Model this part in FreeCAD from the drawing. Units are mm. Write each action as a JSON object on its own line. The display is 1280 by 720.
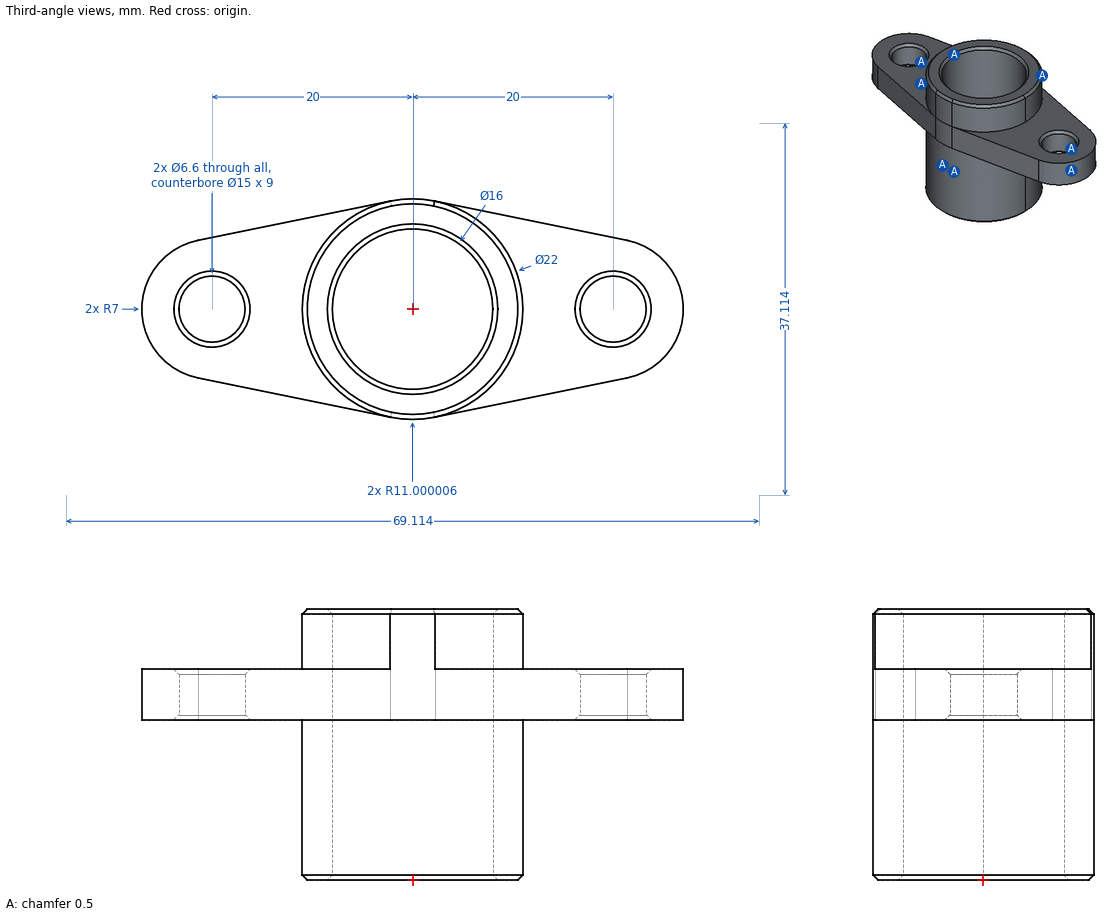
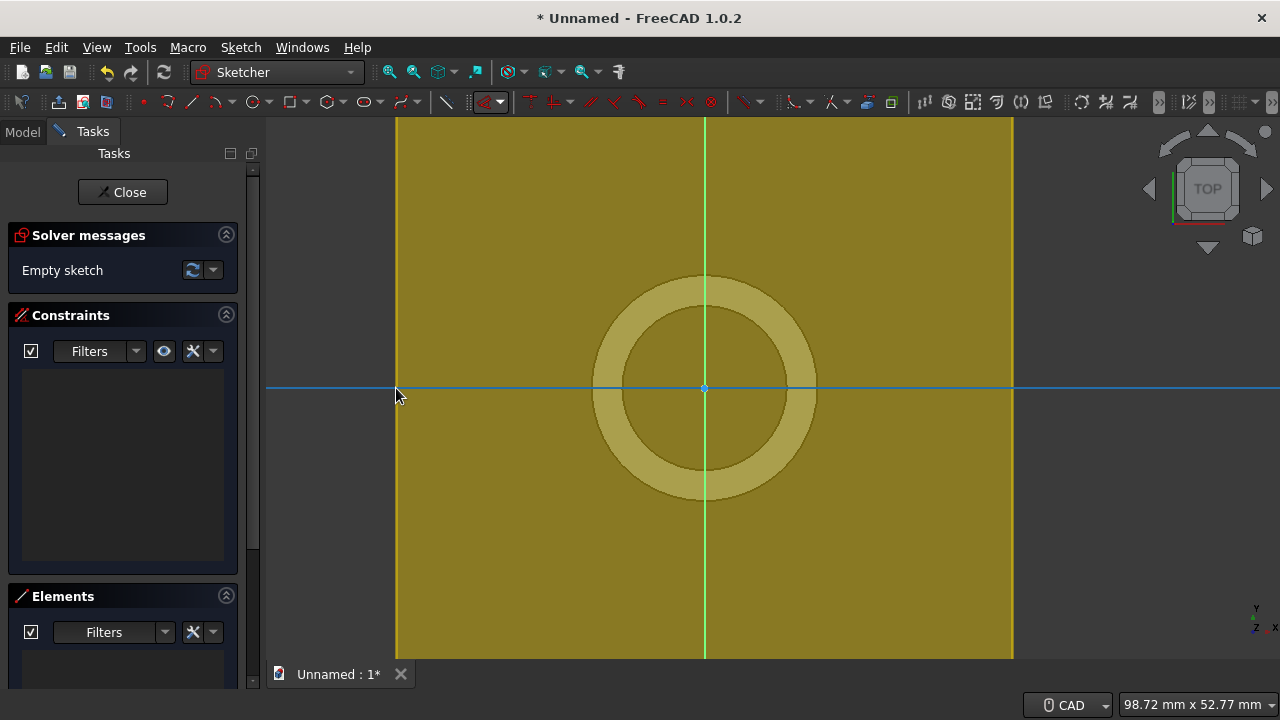
{"action": "left_click", "coordinate": [192, 102]}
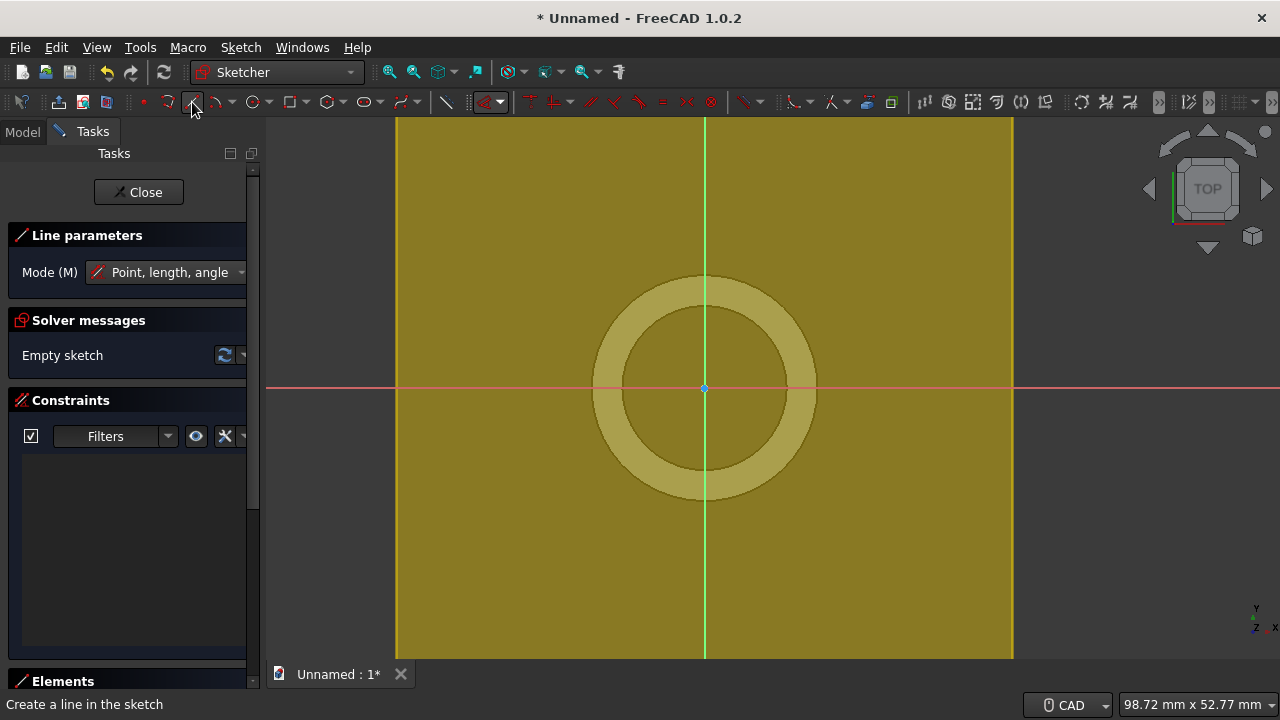
{"action": "left_click", "coordinate": [682, 277]}
{"action": "left_click", "coordinate": [485, 318]}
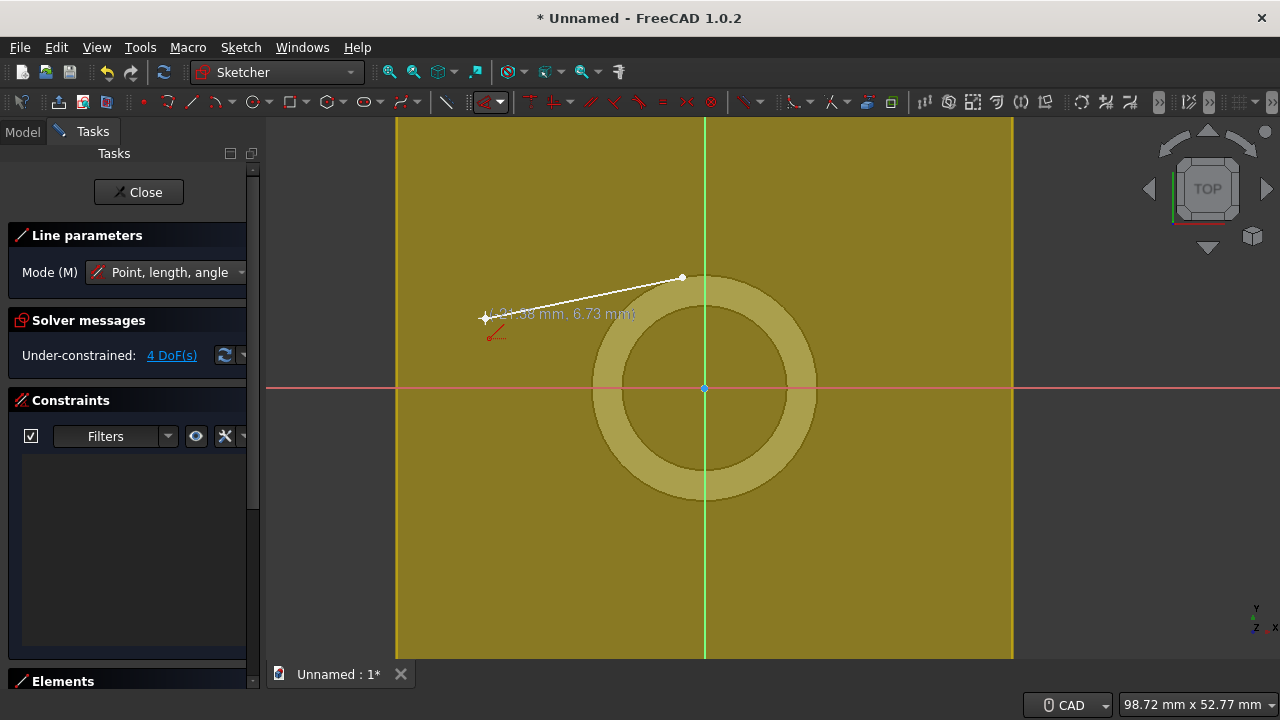
{"action": "left_click", "coordinate": [485, 459]}
{"action": "left_click", "coordinate": [682, 499]}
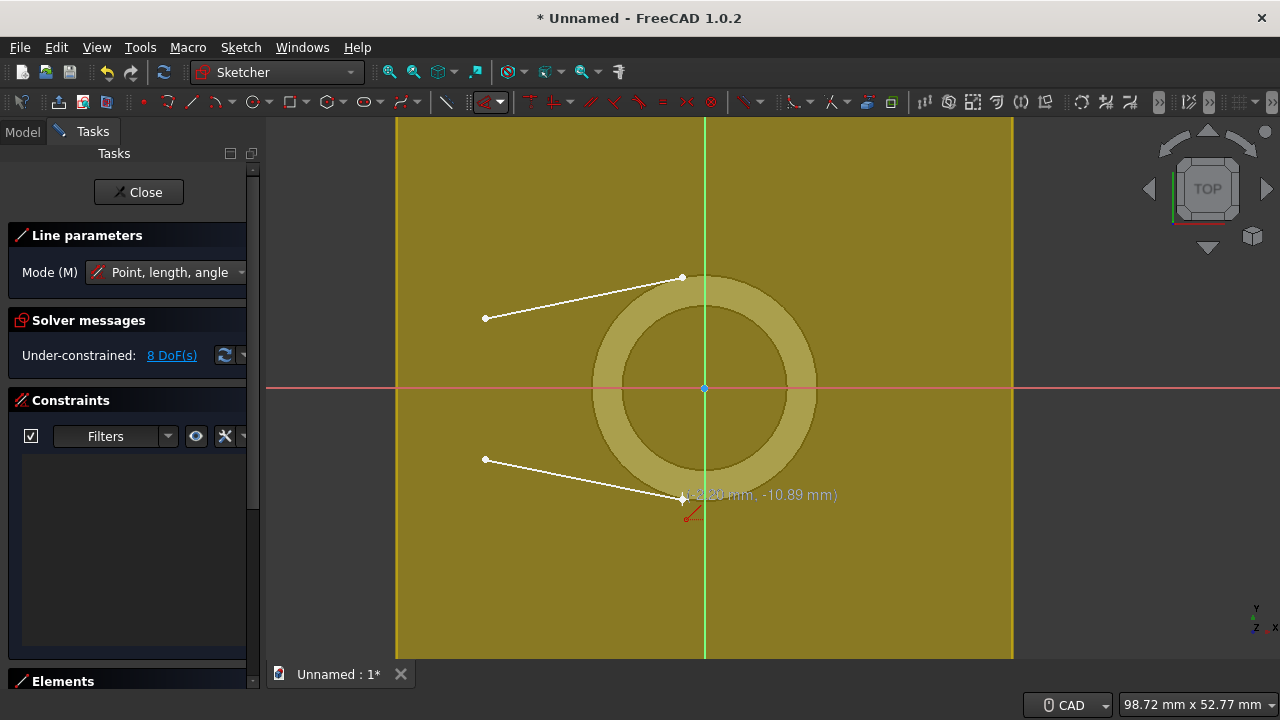
{"action": "left_click", "coordinate": [727, 499]}
{"action": "left_click", "coordinate": [924, 459]}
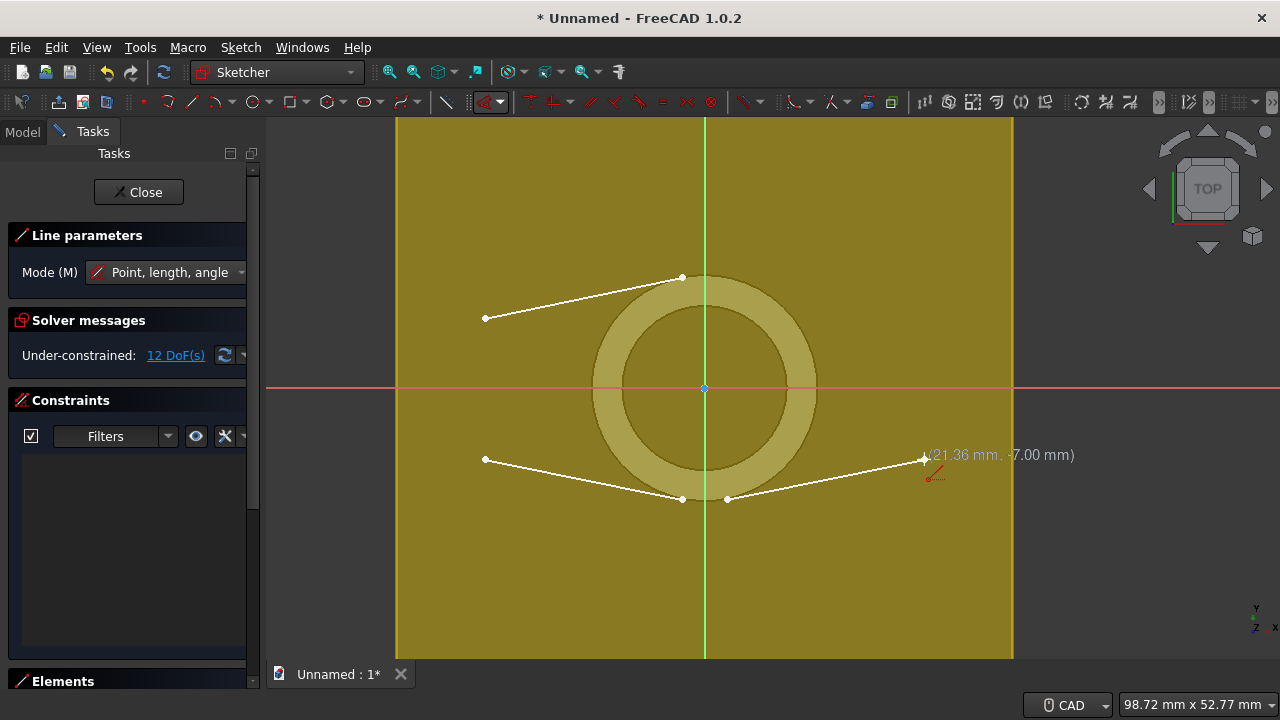
{"action": "left_click", "coordinate": [924, 318]}
{"action": "left_click", "coordinate": [727, 277]}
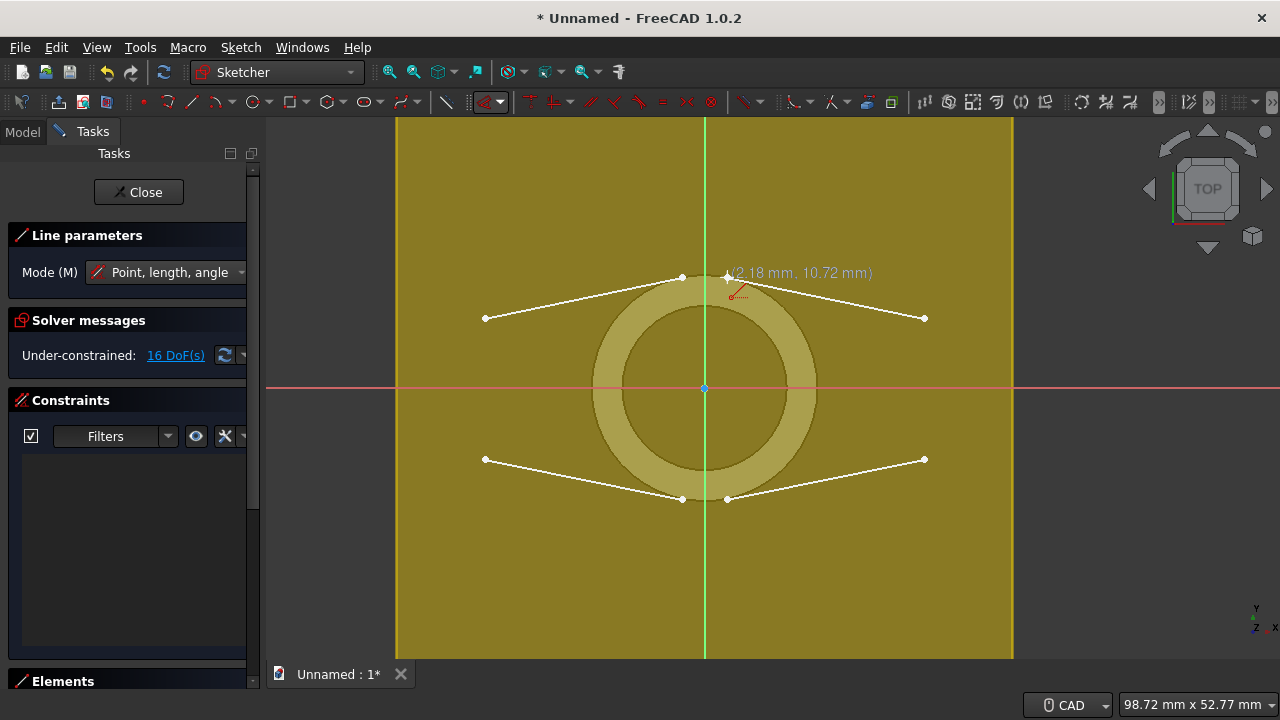
{"action": "left_click", "coordinate": [234, 102]}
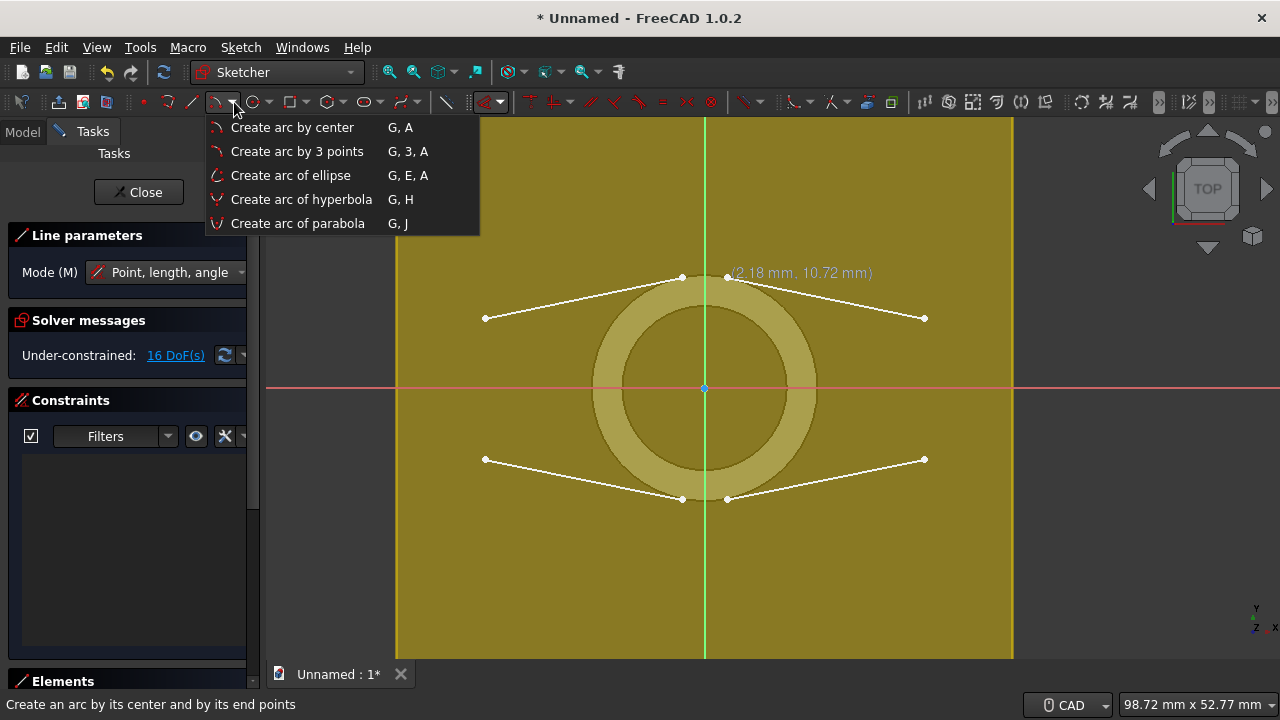
{"action": "left_click", "coordinate": [342, 151]}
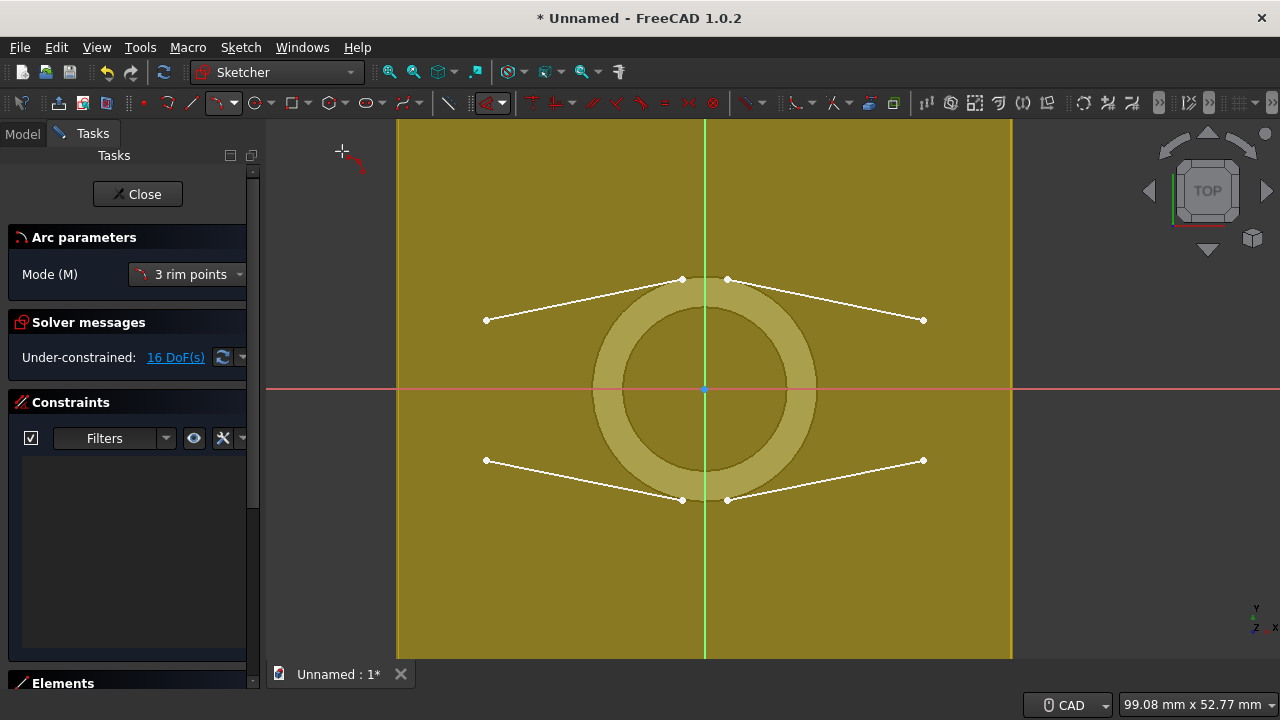
{"action": "left_click", "coordinate": [486, 320]}
{"action": "left_click", "coordinate": [486, 461]}
{"action": "left_click", "coordinate": [431, 370]}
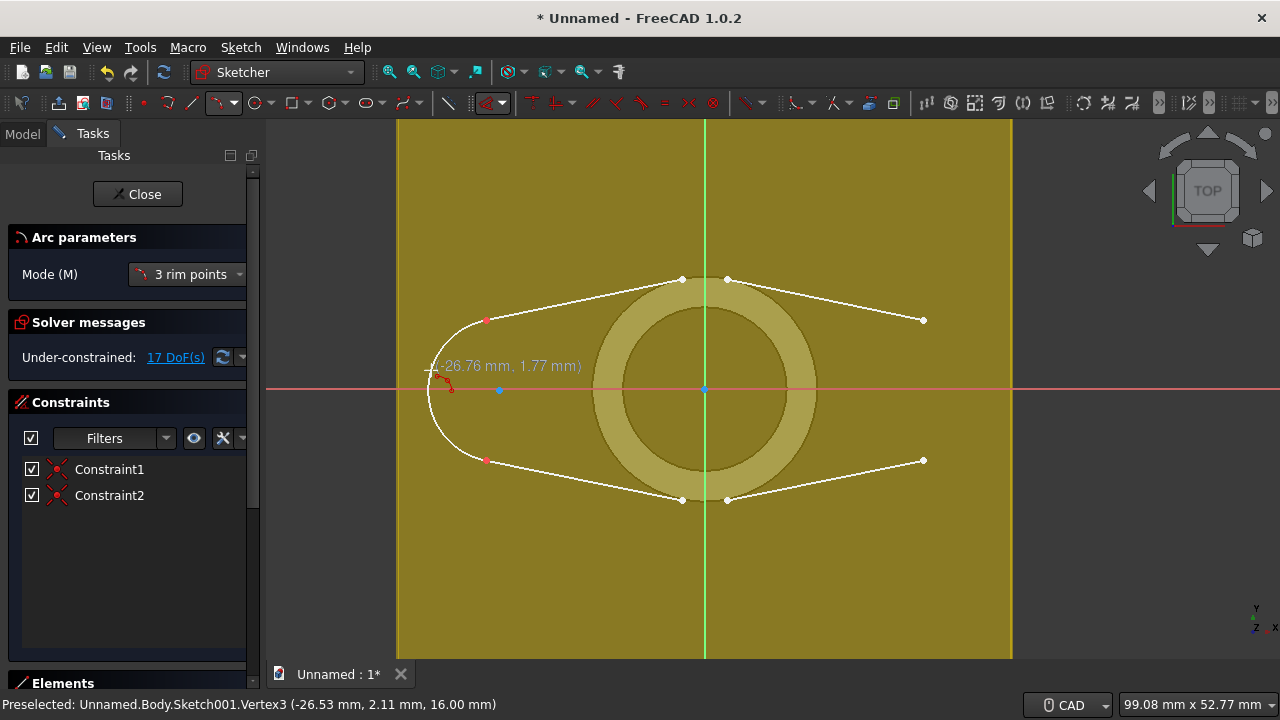
{"action": "left_click", "coordinate": [682, 501]}
{"action": "left_click", "coordinate": [727, 501]}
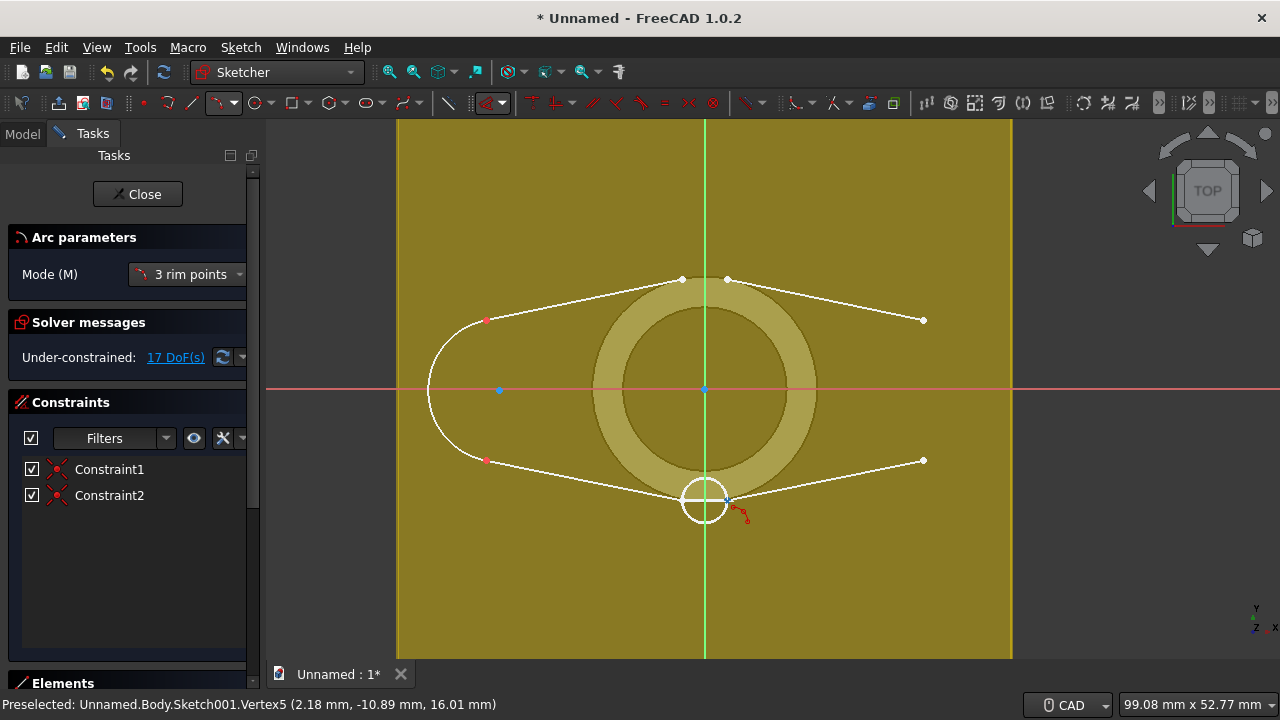
{"action": "scroll", "coordinate": [700, 502], "scroll_direction": "up", "scroll_amount": 10}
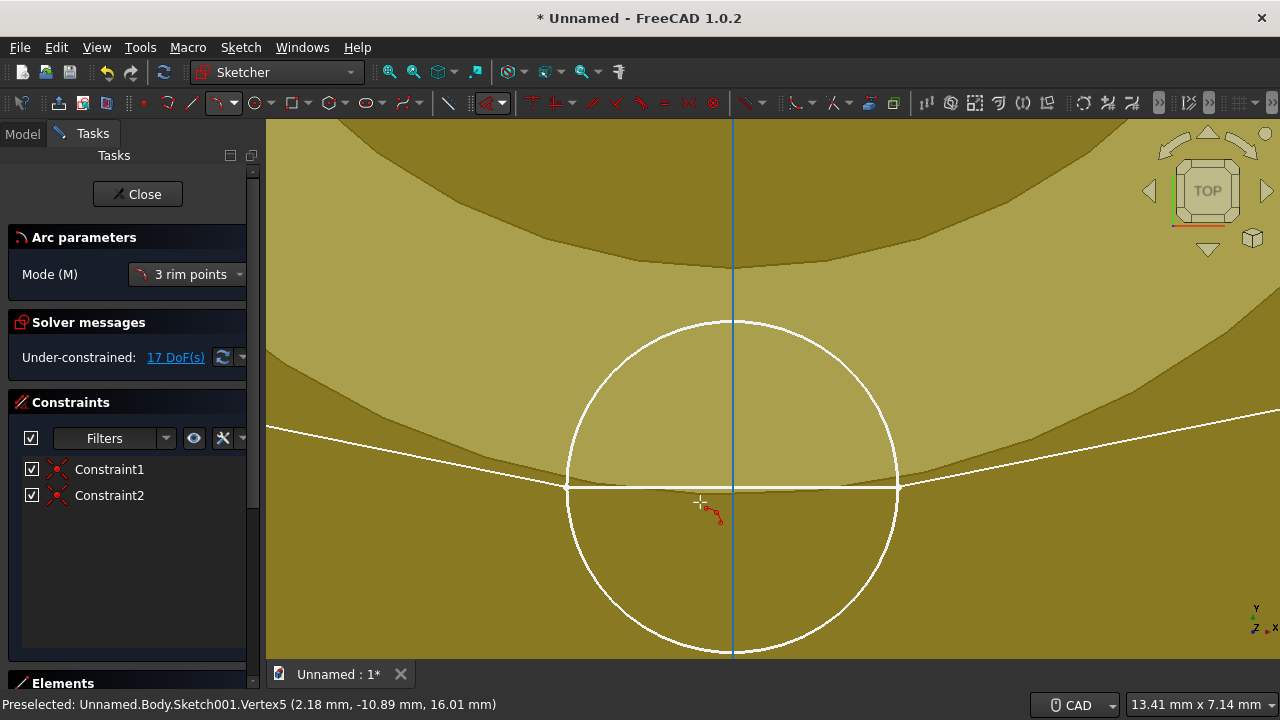
{"action": "left_click", "coordinate": [699, 494]}